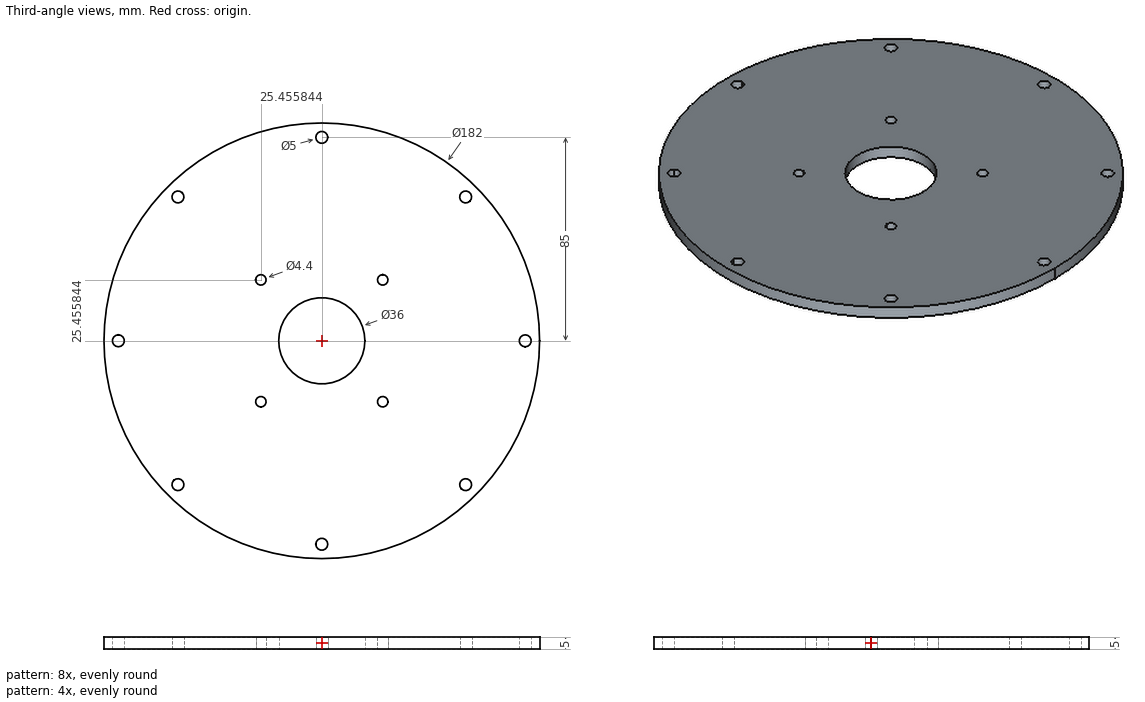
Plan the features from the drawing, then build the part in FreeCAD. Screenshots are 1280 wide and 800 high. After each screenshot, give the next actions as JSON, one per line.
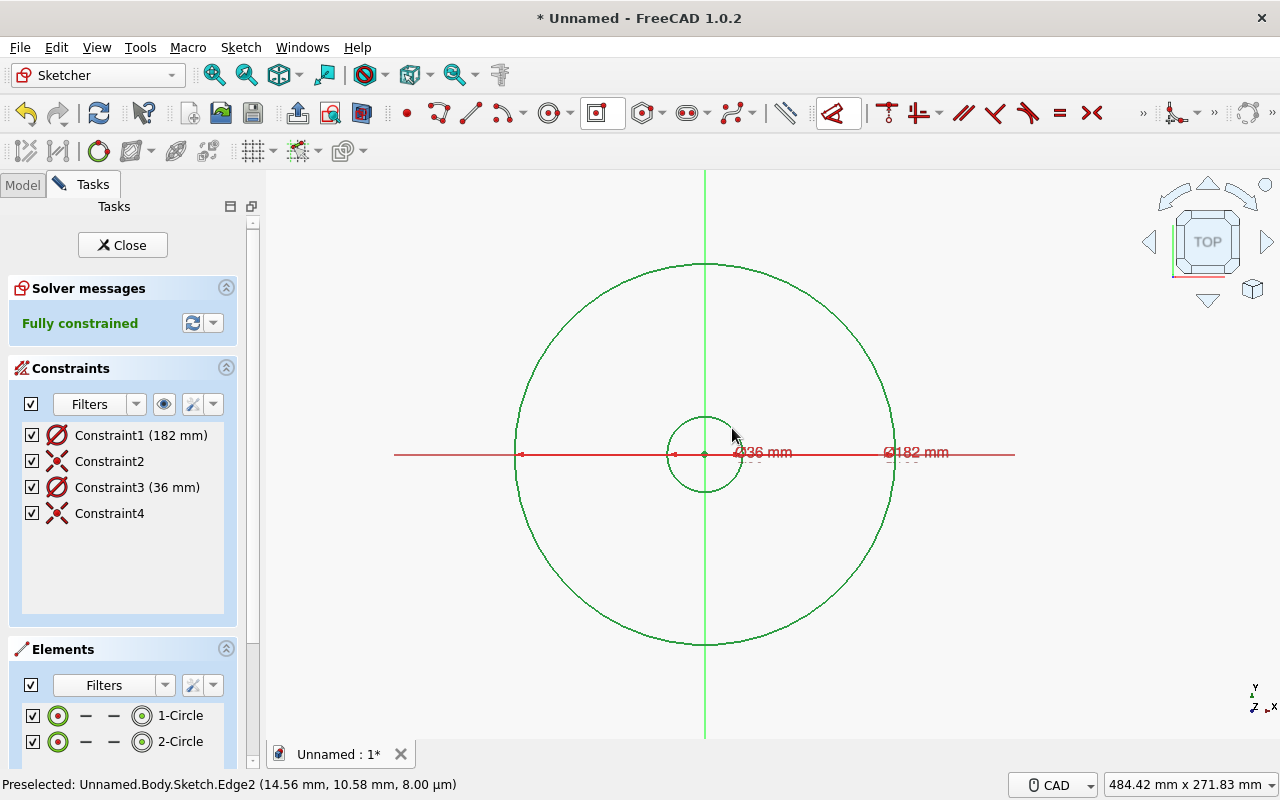
{"action": "left_click", "coordinate": [123, 245]}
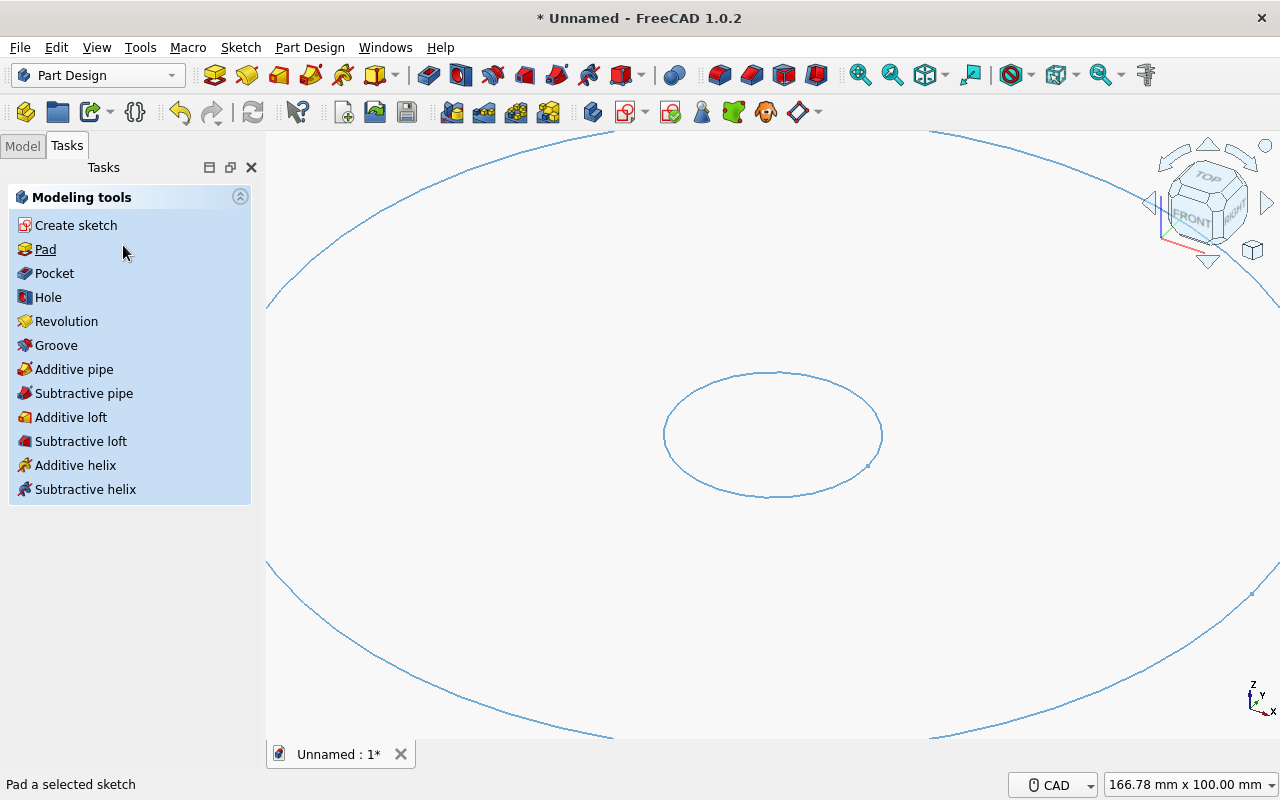
{"action": "left_click", "coordinate": [216, 76]}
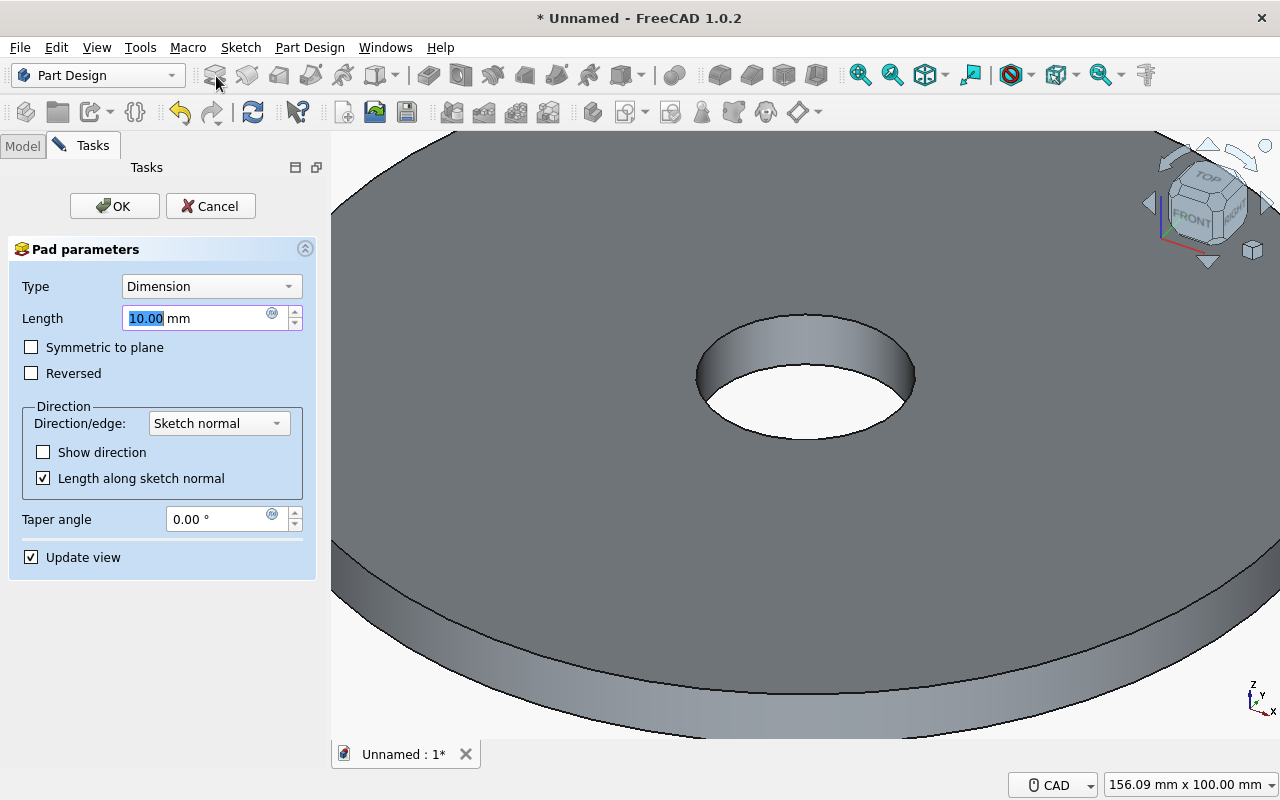
{"action": "type", "text": "5"}
{"action": "key", "text": "Tab"}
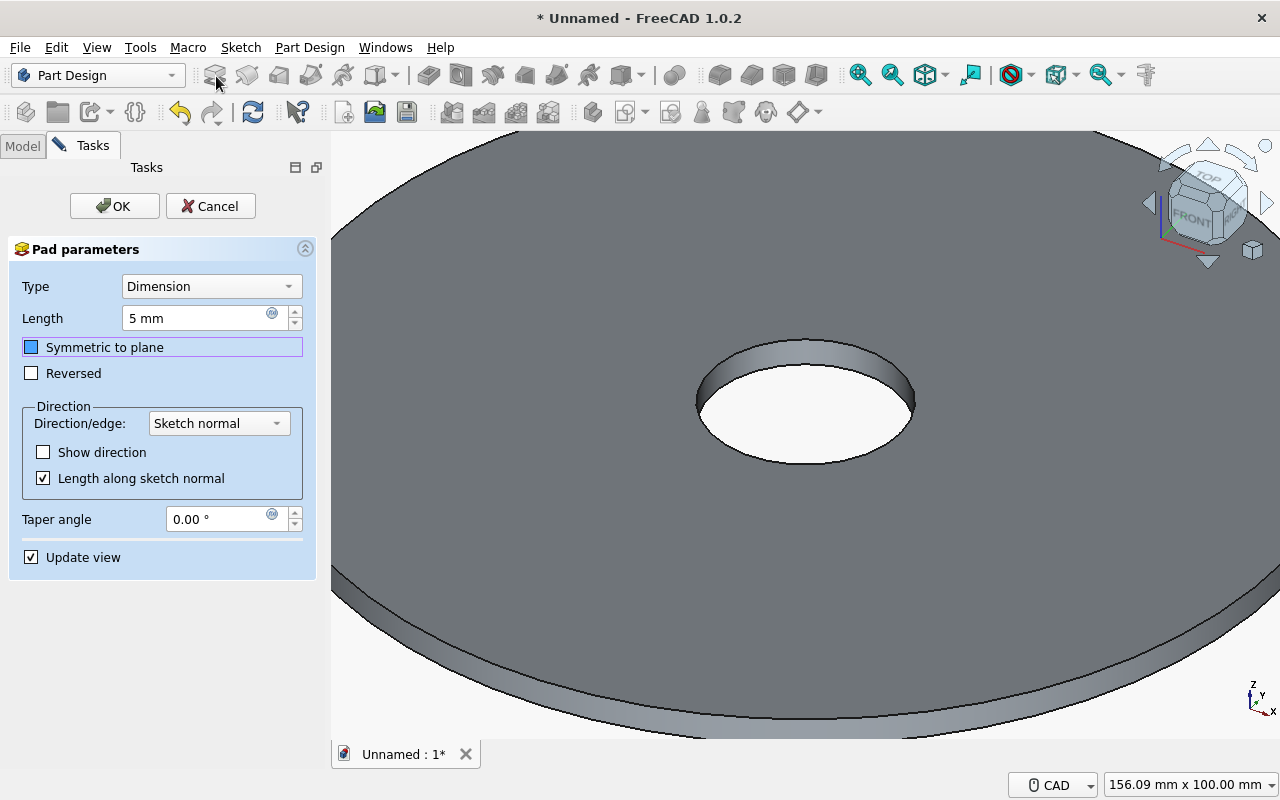
{"action": "left_click", "coordinate": [30, 347]}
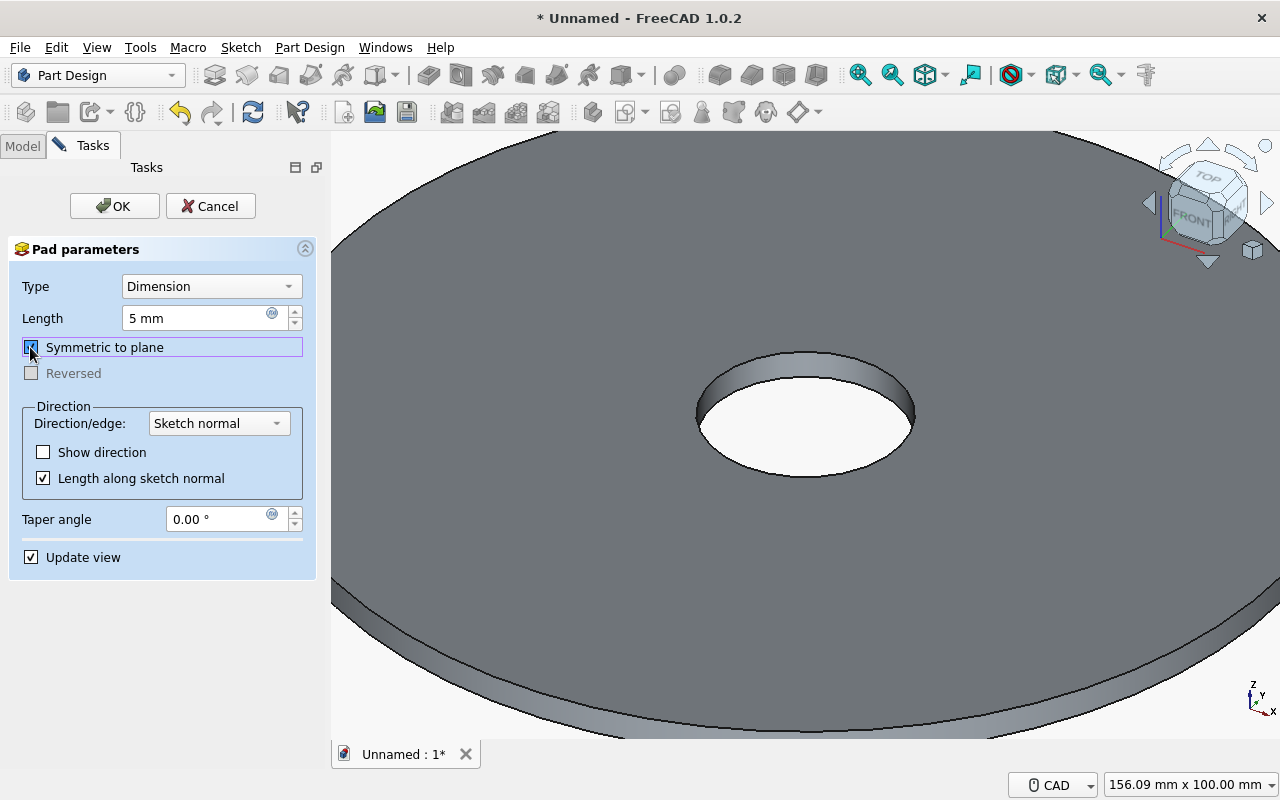
{"action": "left_click", "coordinate": [115, 206]}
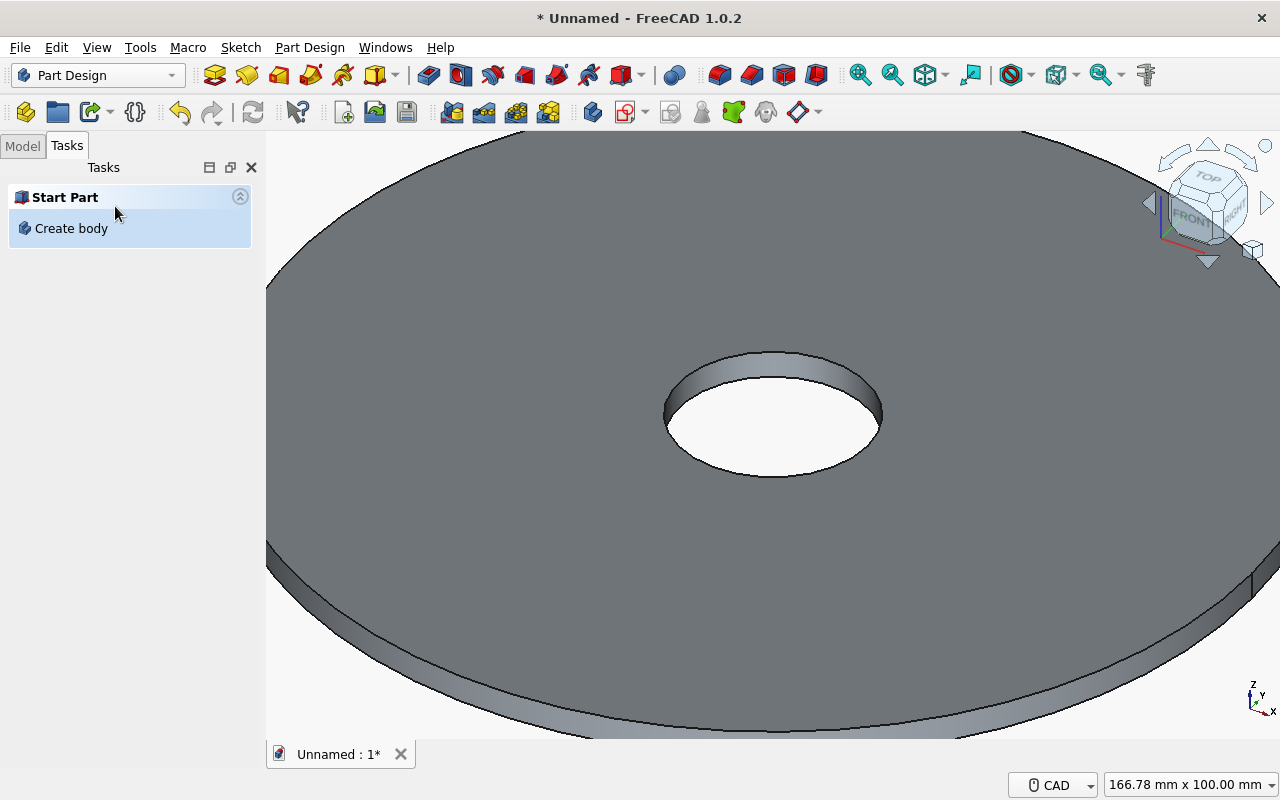
{"action": "left_click", "coordinate": [862, 76]}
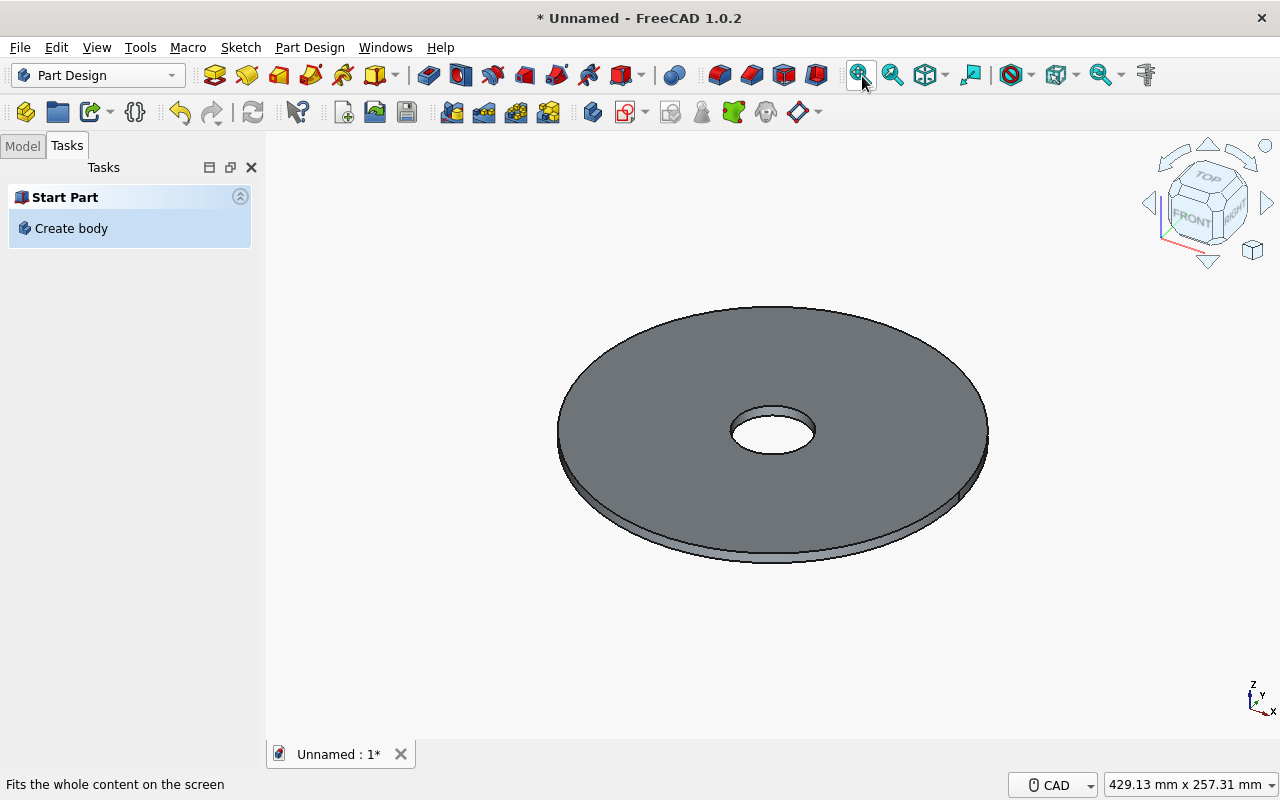
{"action": "left_click", "coordinate": [834, 368]}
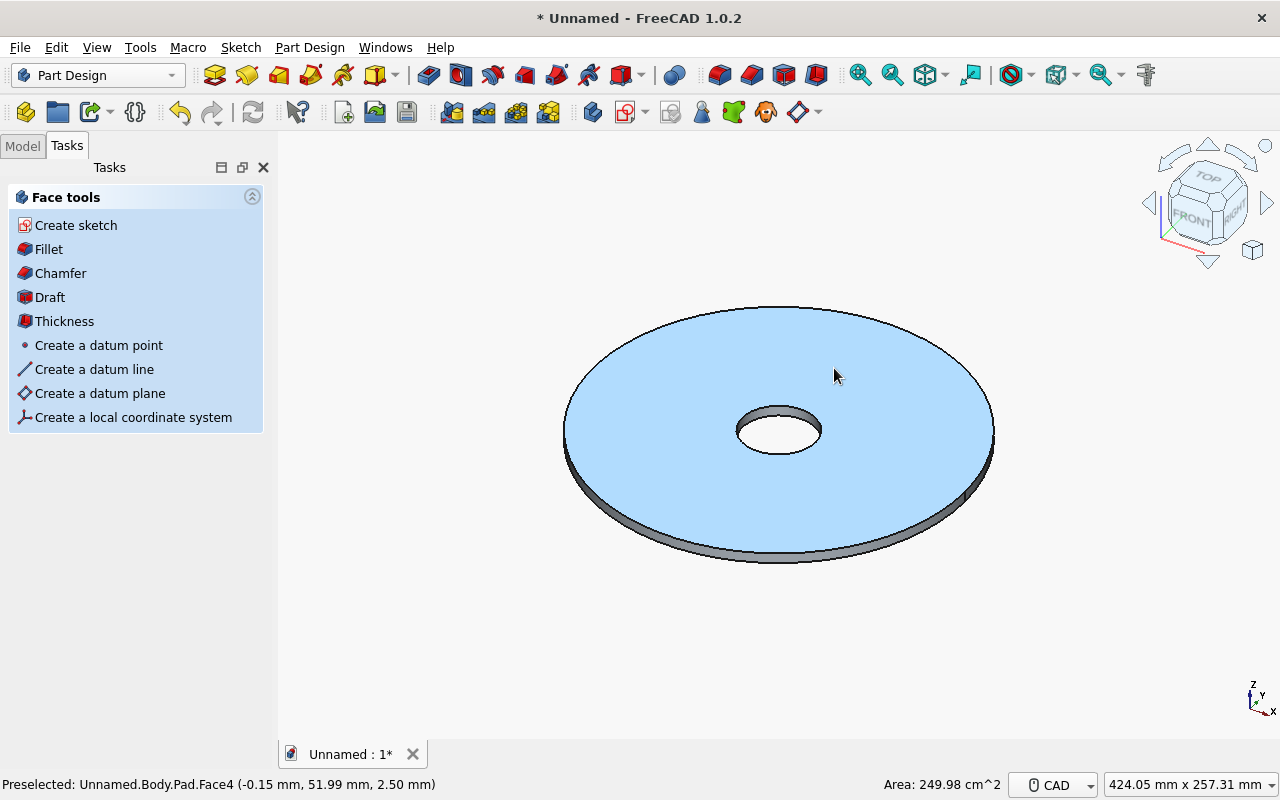
{"action": "left_click", "coordinate": [626, 112]}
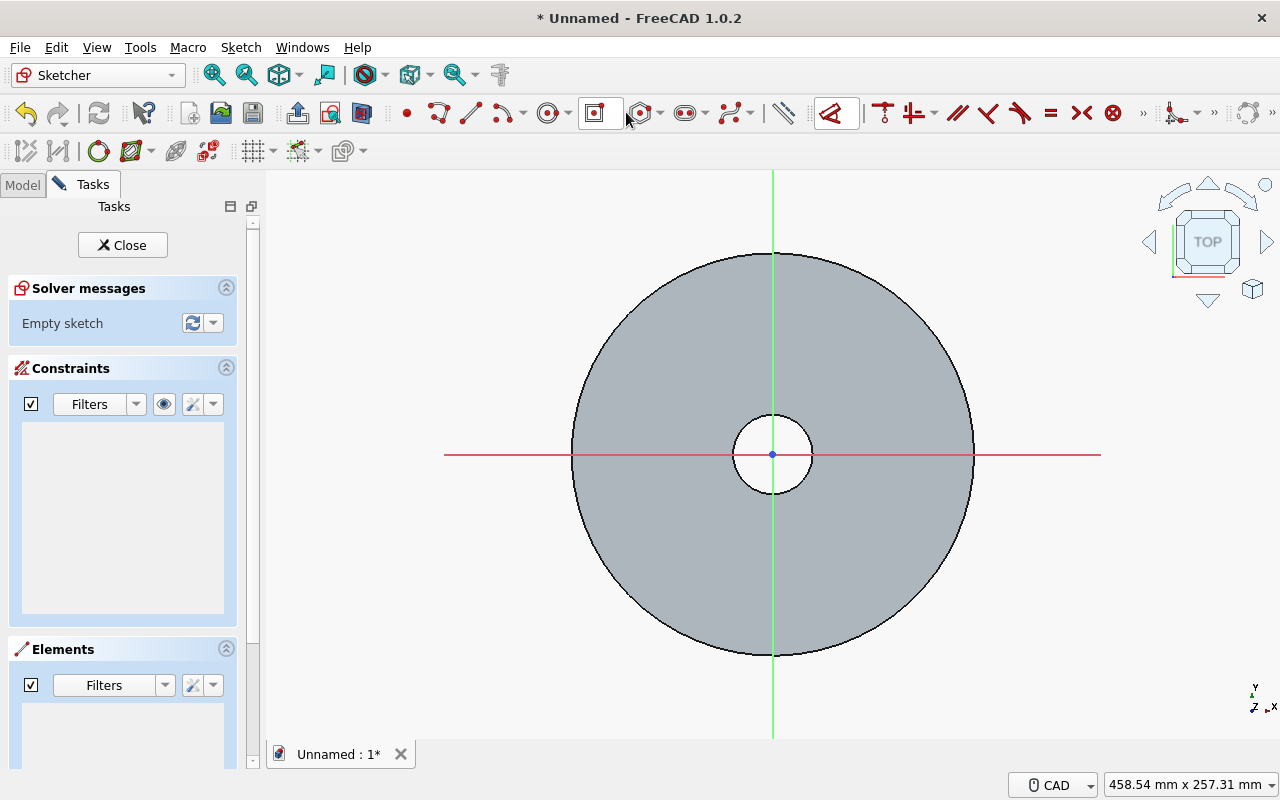
{"action": "scroll", "coordinate": [776, 257], "scroll_direction": "up", "scroll_amount": 15}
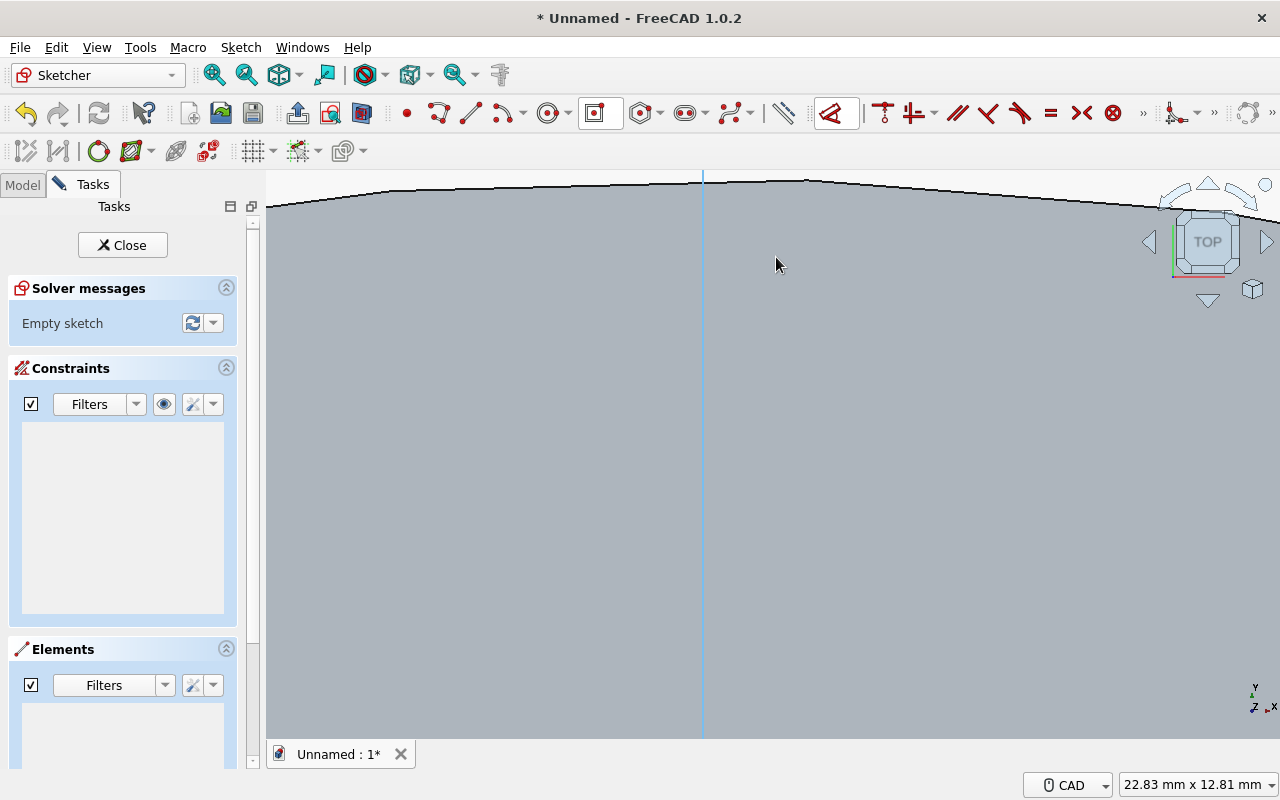
{"action": "scroll", "coordinate": [701, 427], "scroll_direction": "up", "scroll_amount": 2}